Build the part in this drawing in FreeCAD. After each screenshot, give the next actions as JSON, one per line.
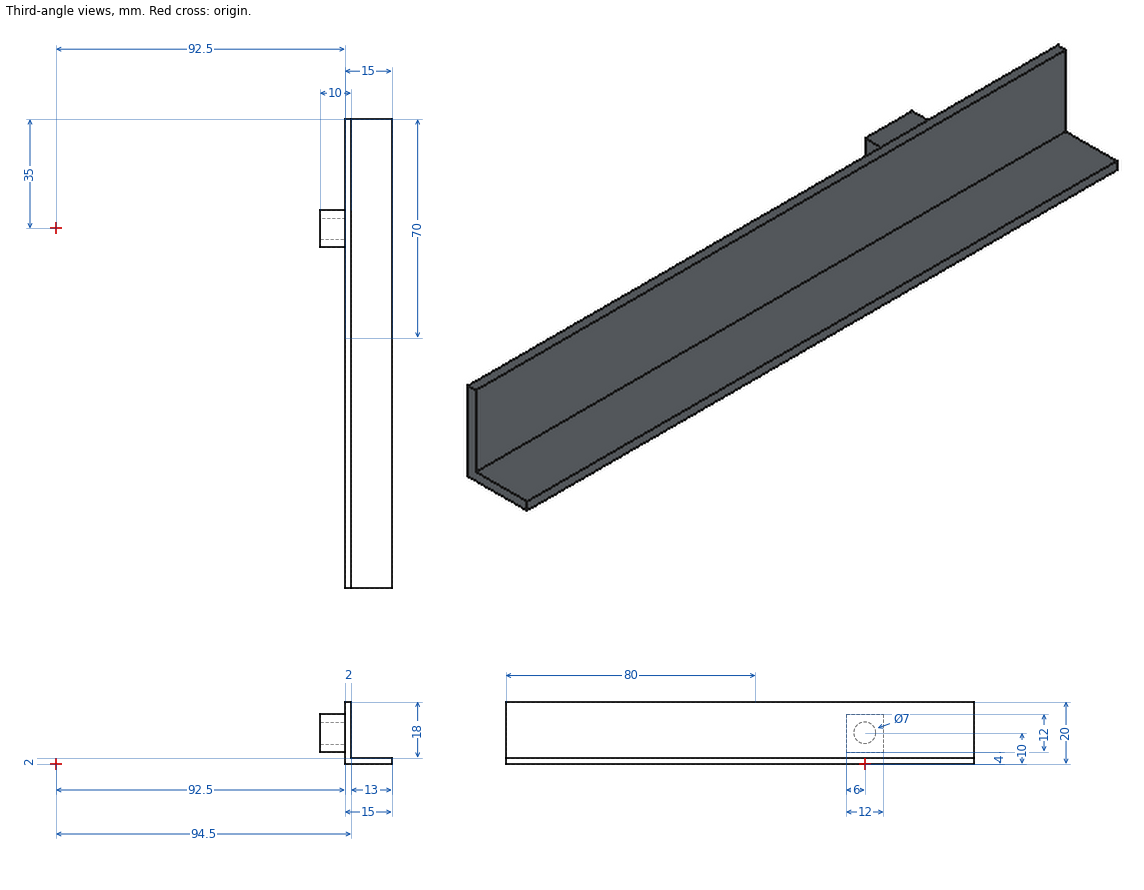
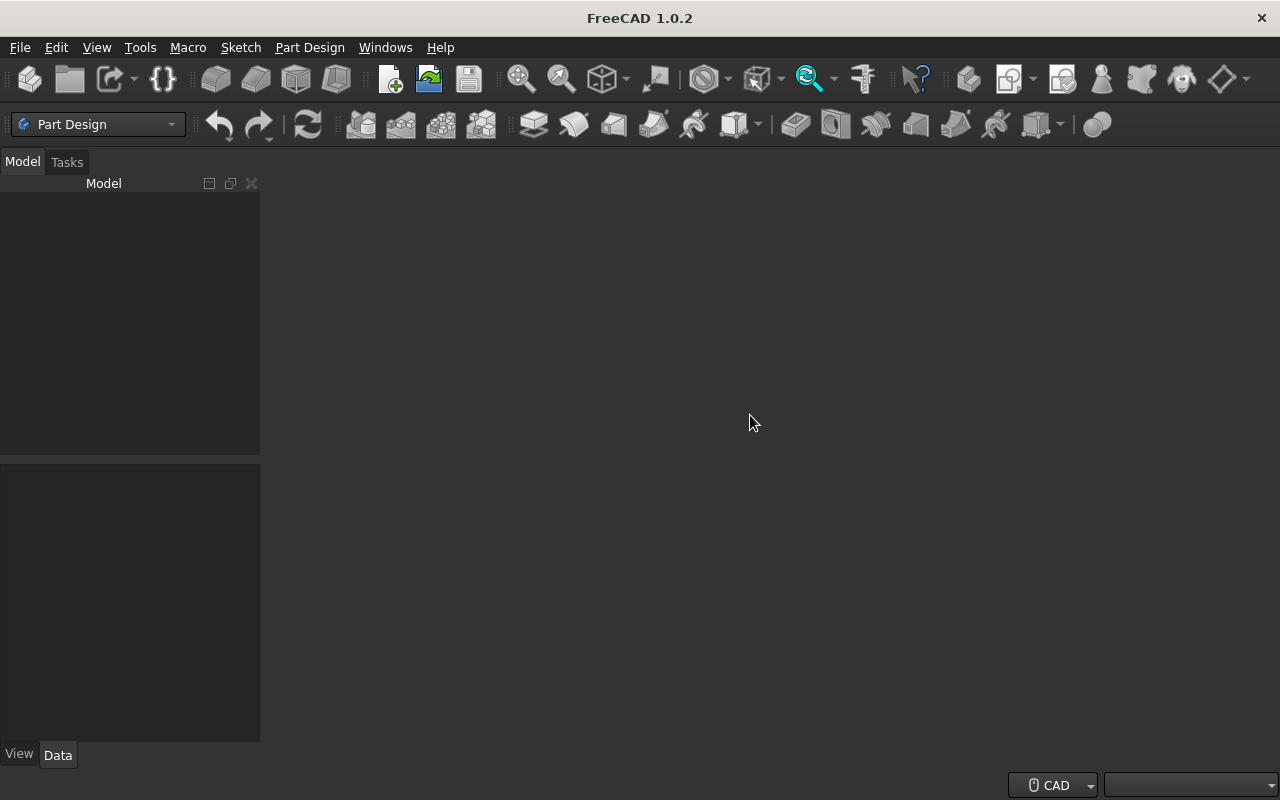
{"action": "left_click", "coordinate": [390, 80]}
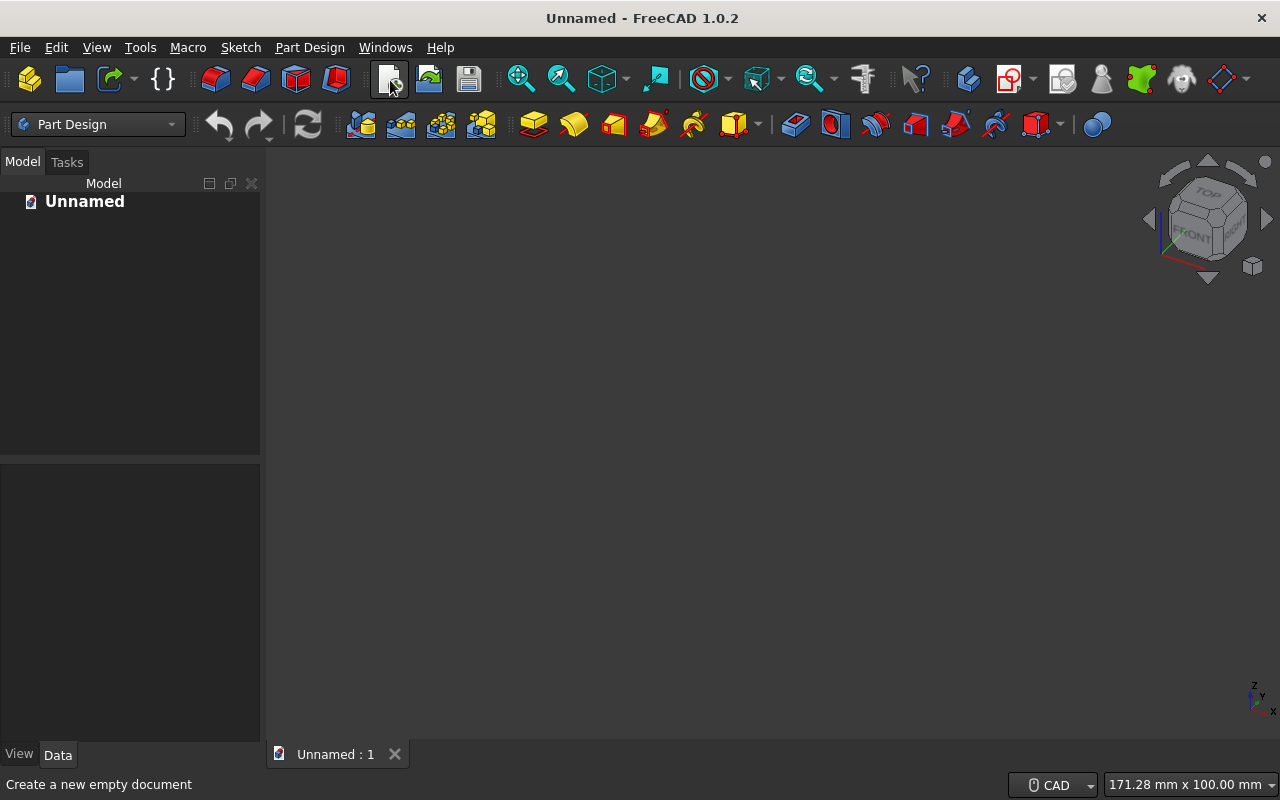
{"action": "left_click", "coordinate": [1010, 80]}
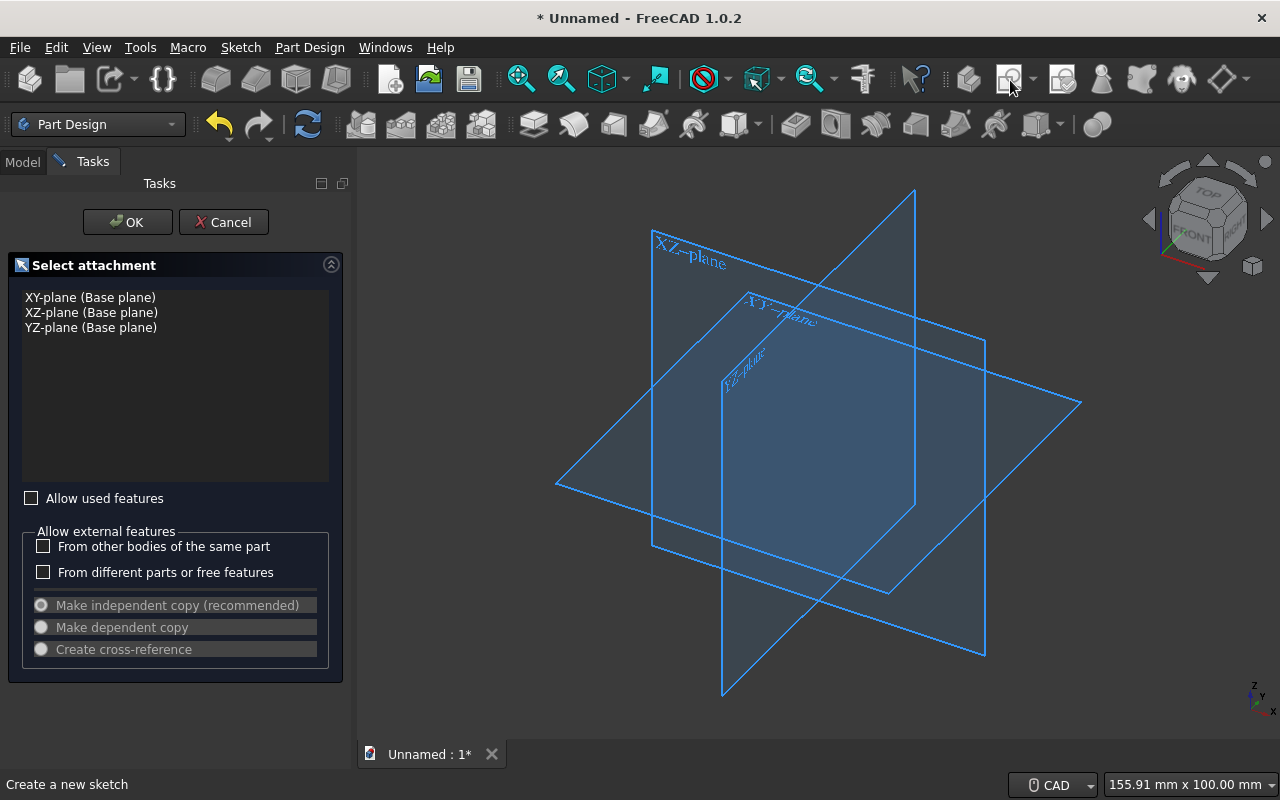
{"action": "left_click", "coordinate": [82, 298]}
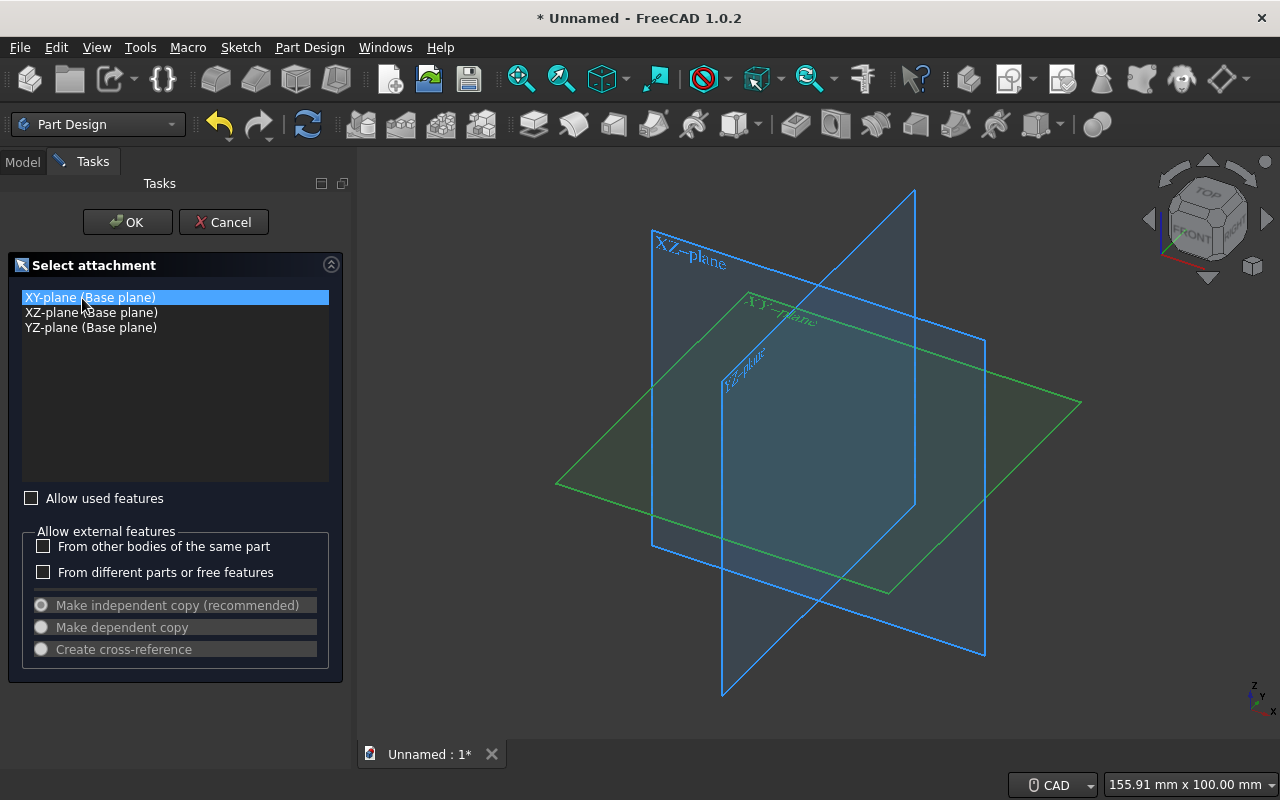
{"action": "left_click", "coordinate": [128, 222]}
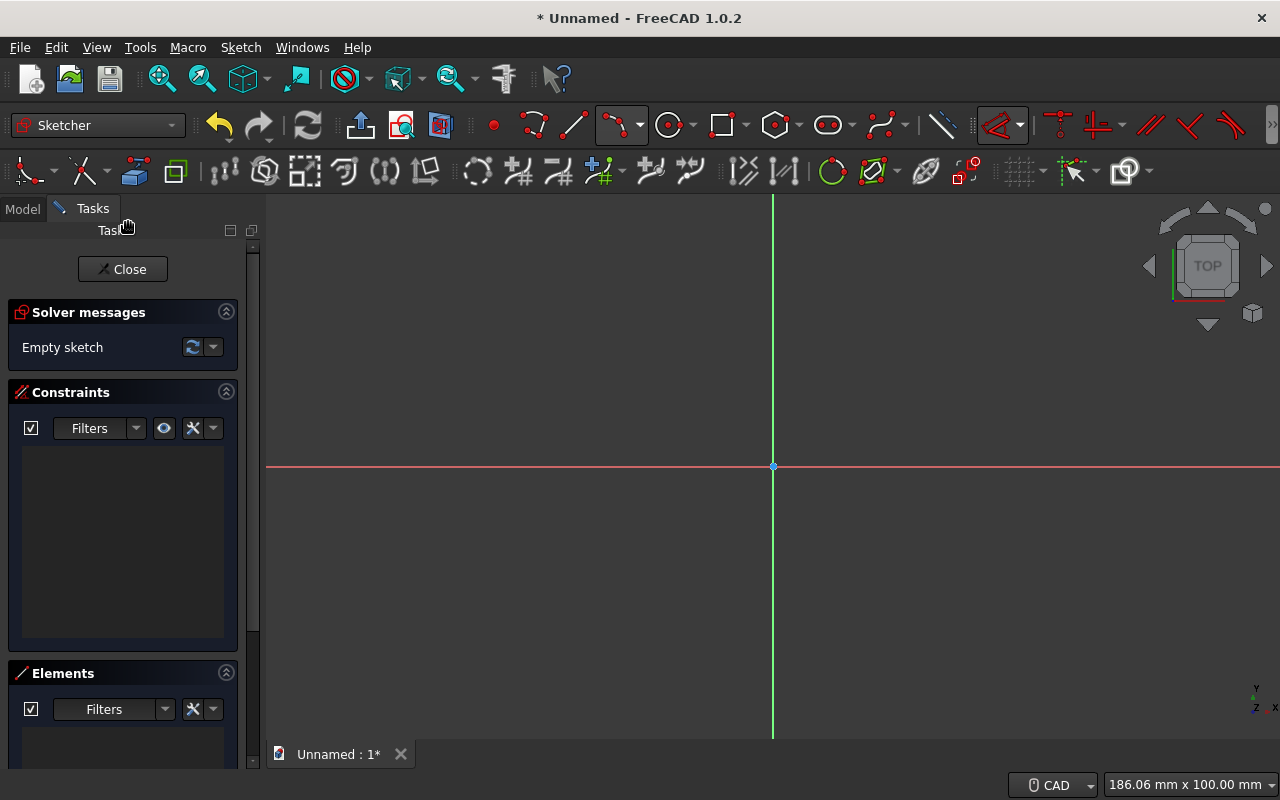
{"action": "scroll", "coordinate": [294, 466], "scroll_direction": "down", "scroll_amount": 2}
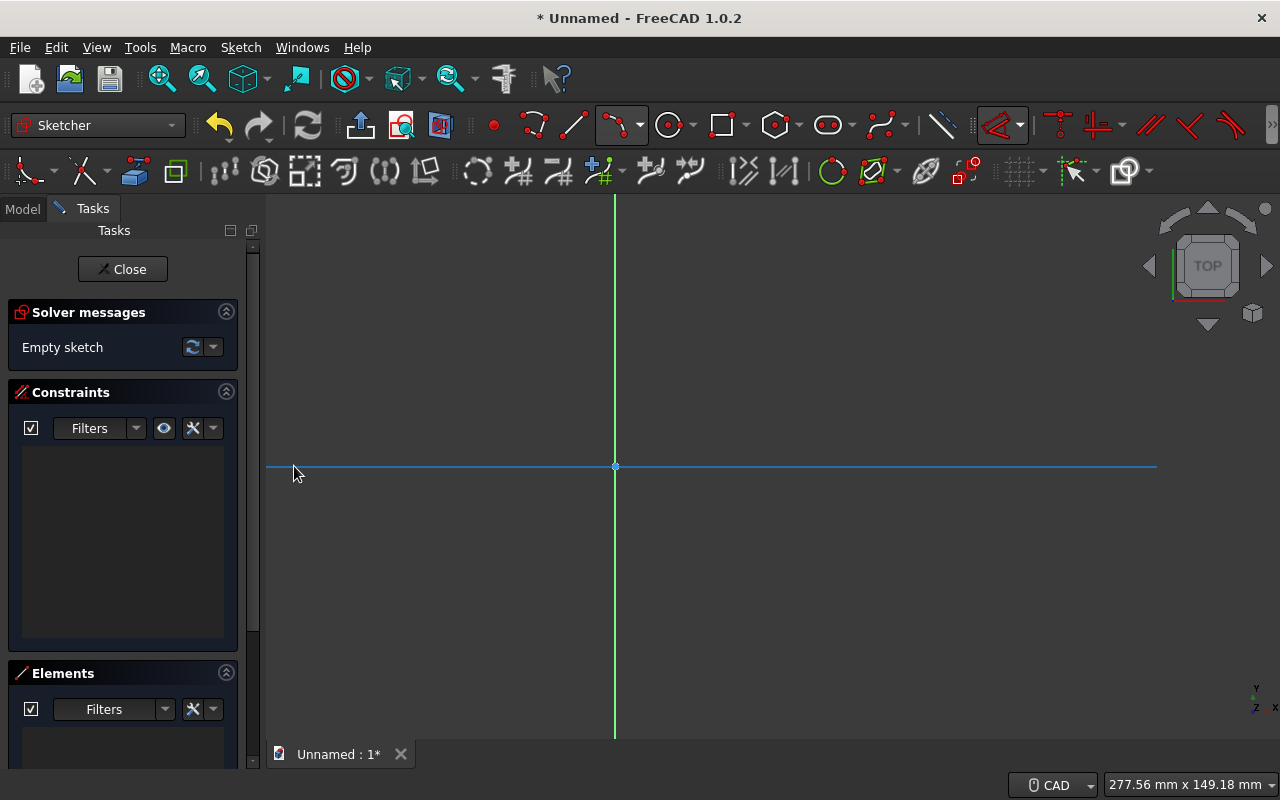
{"action": "left_click", "coordinate": [722, 126]}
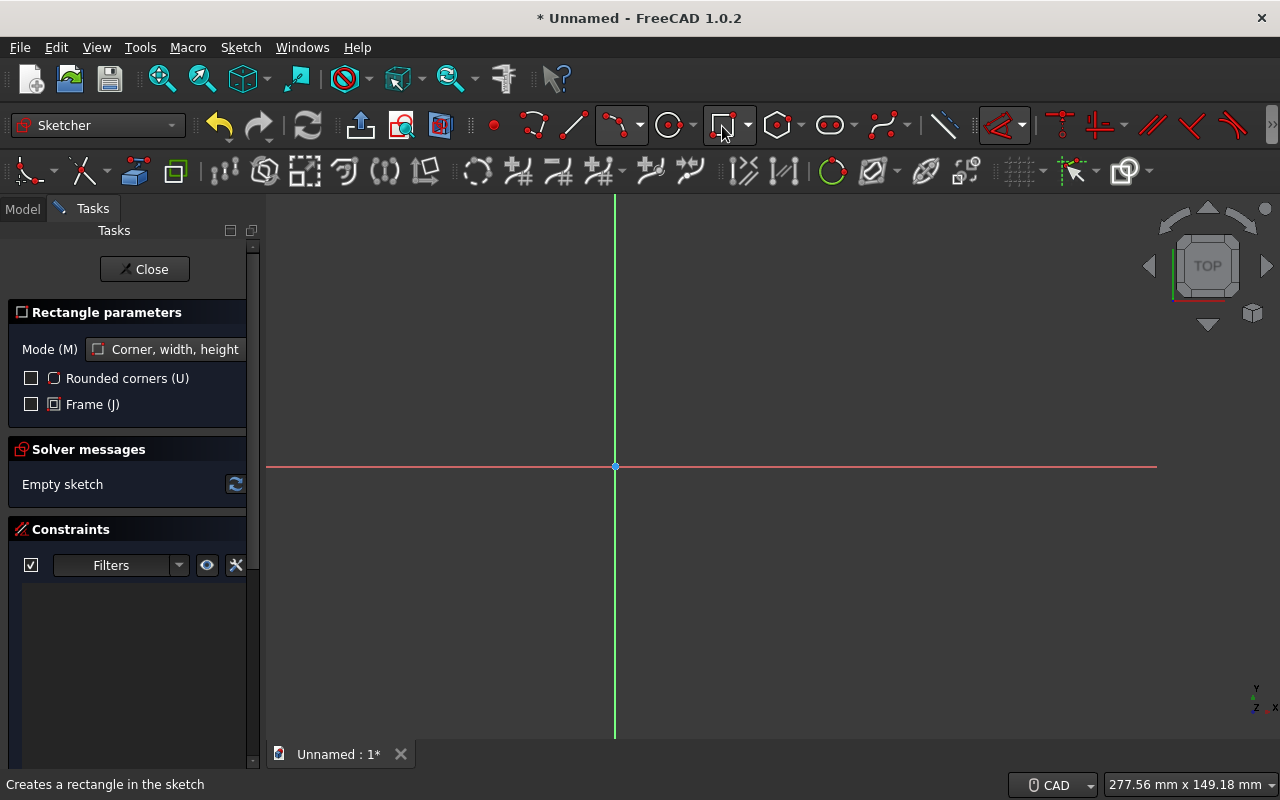
{"action": "left_click", "coordinate": [953, 339]}
{"action": "left_click", "coordinate": [1008, 594]}
{"action": "key", "text": "Escape"}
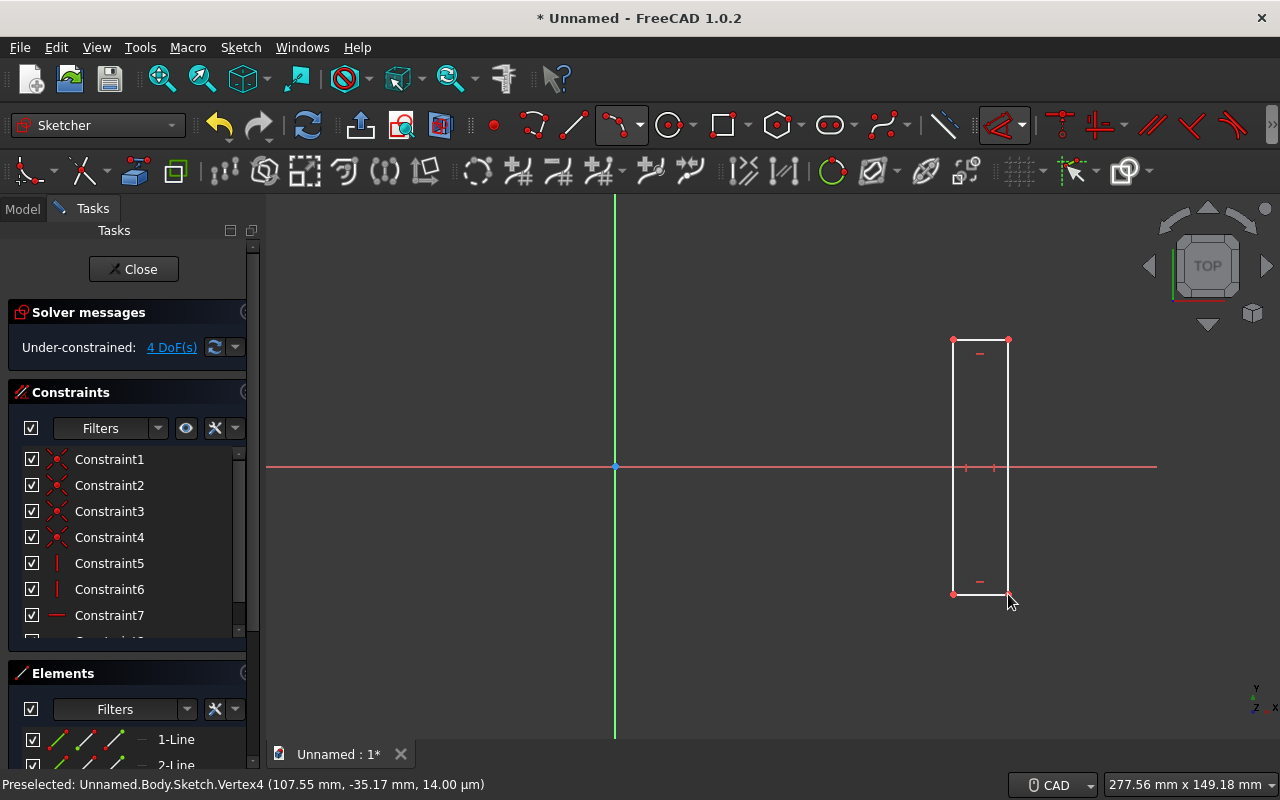
{"action": "left_click", "coordinate": [953, 417]}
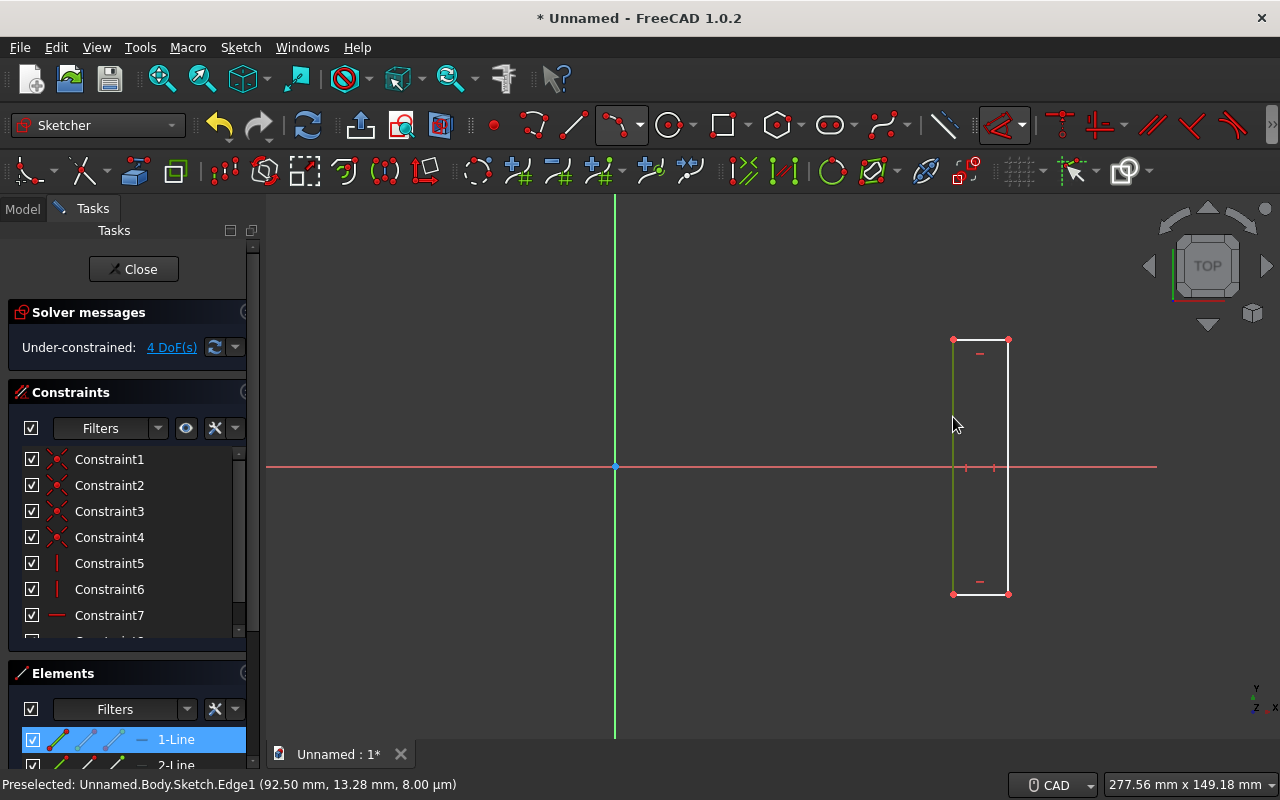
{"action": "left_click", "coordinate": [1024, 126]}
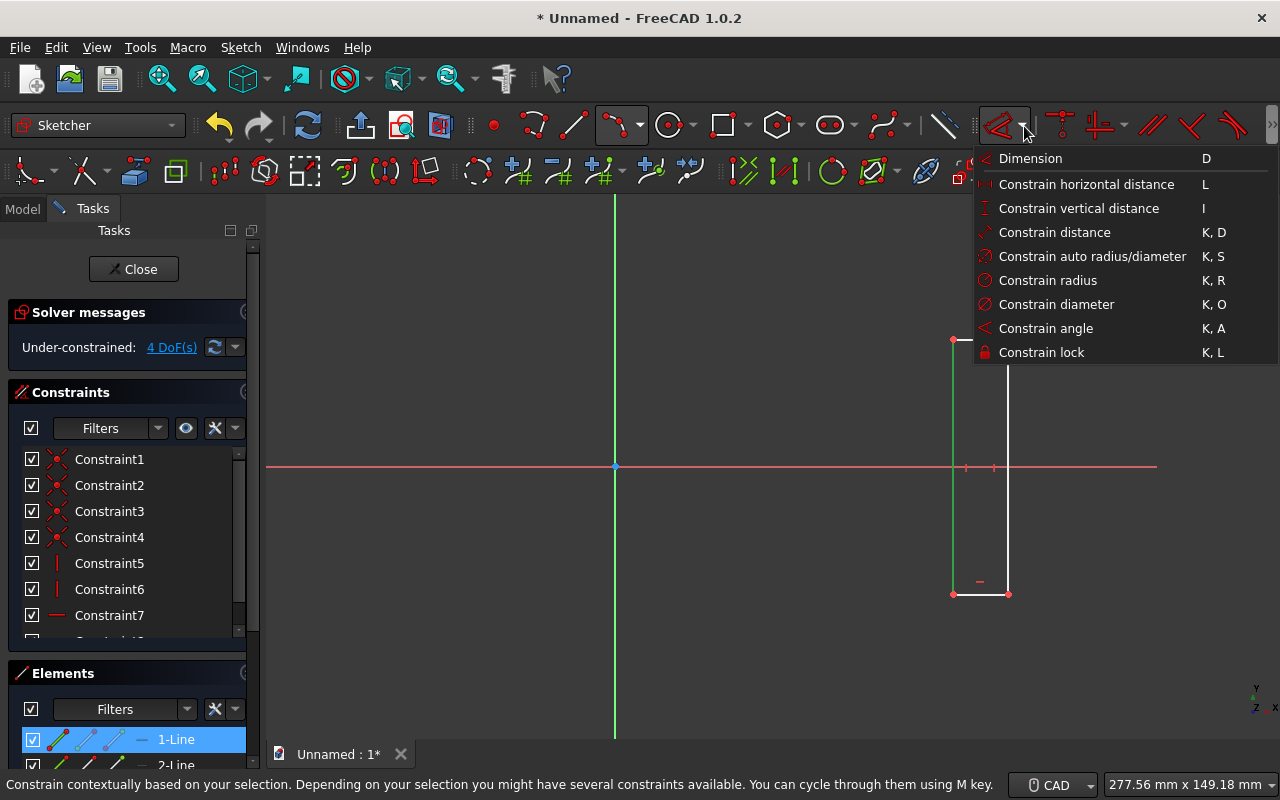
{"action": "left_click", "coordinate": [1126, 208]}